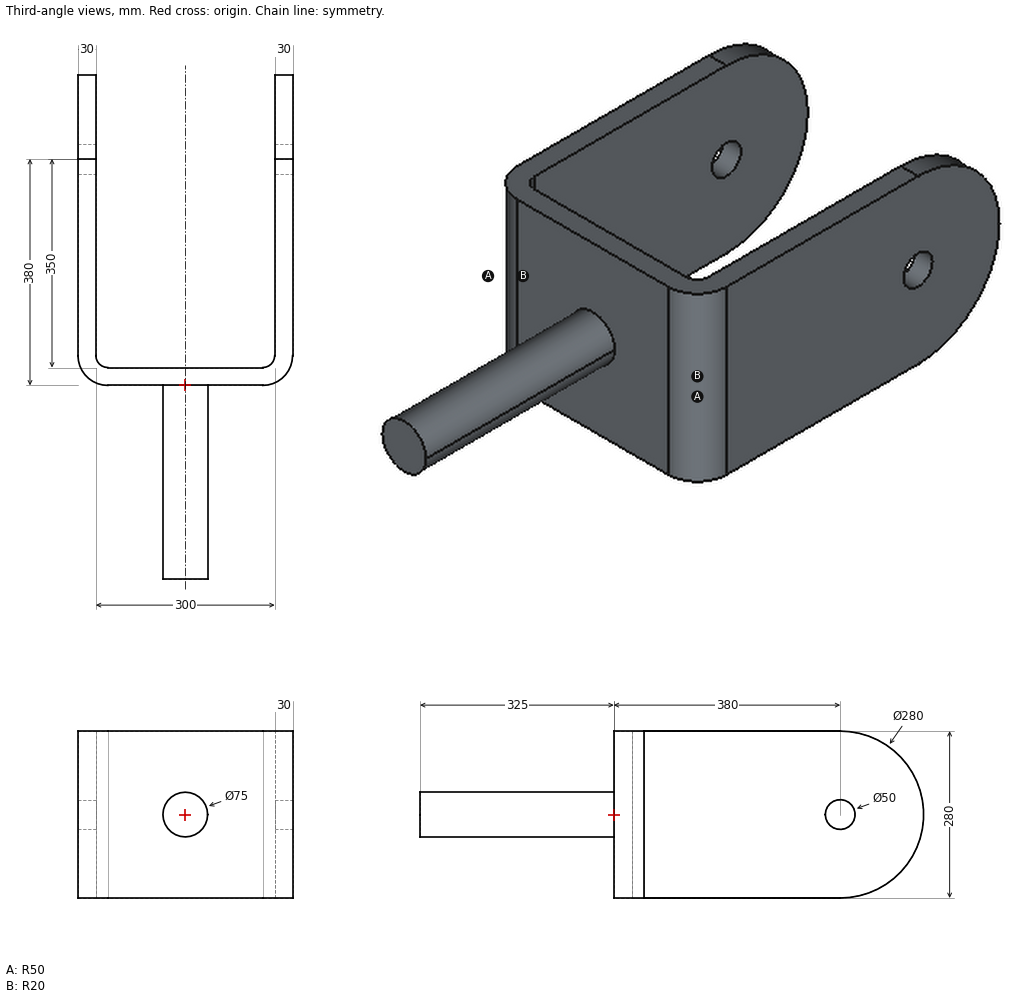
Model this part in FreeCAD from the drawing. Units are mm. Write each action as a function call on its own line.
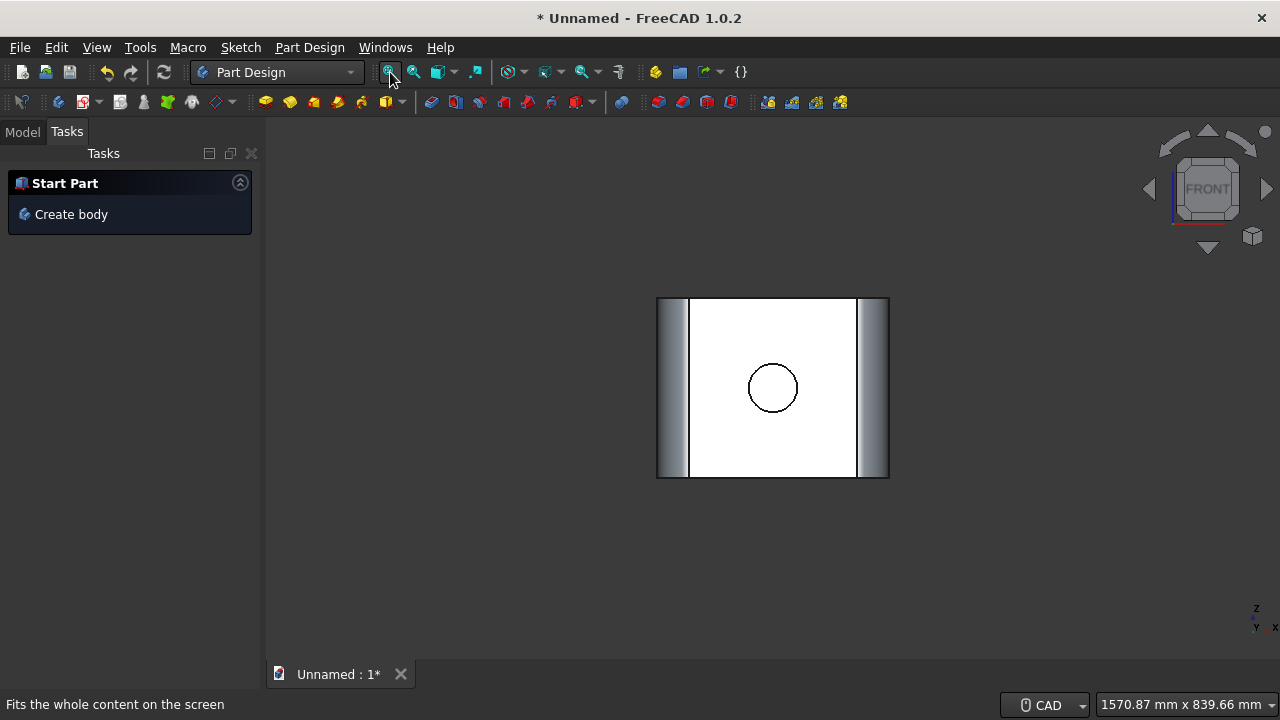
click(390, 72)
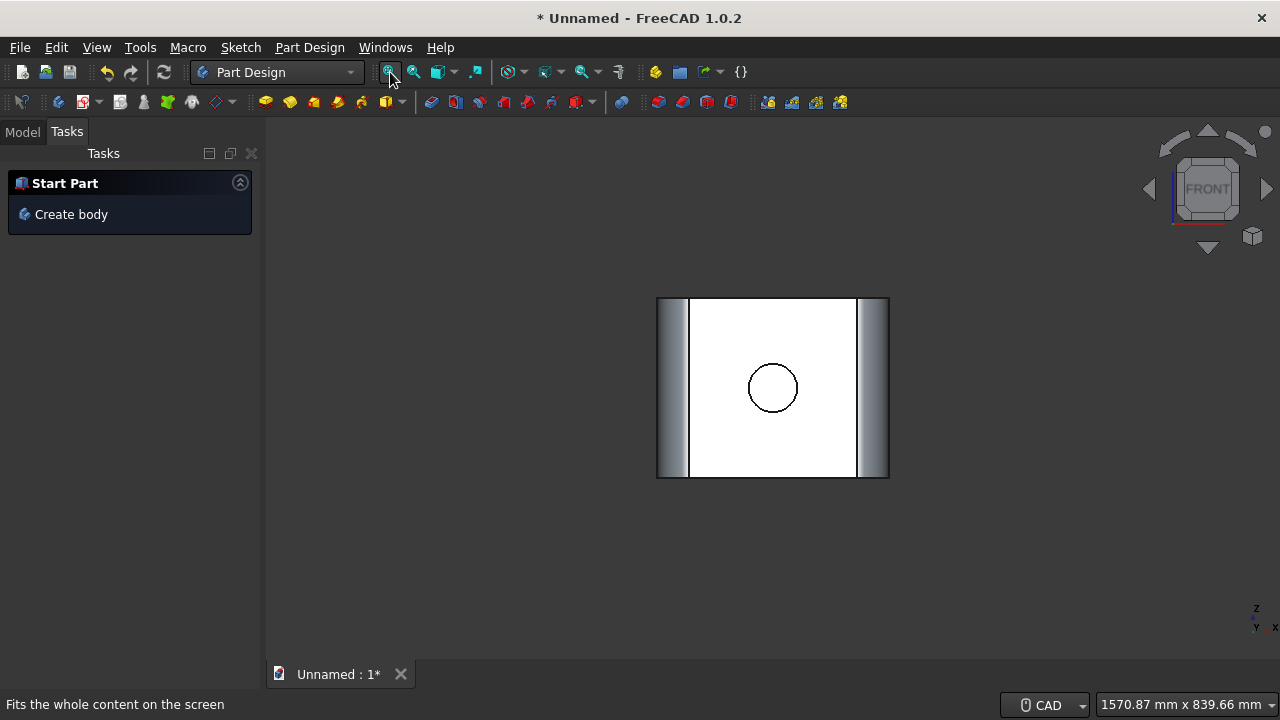
key(3)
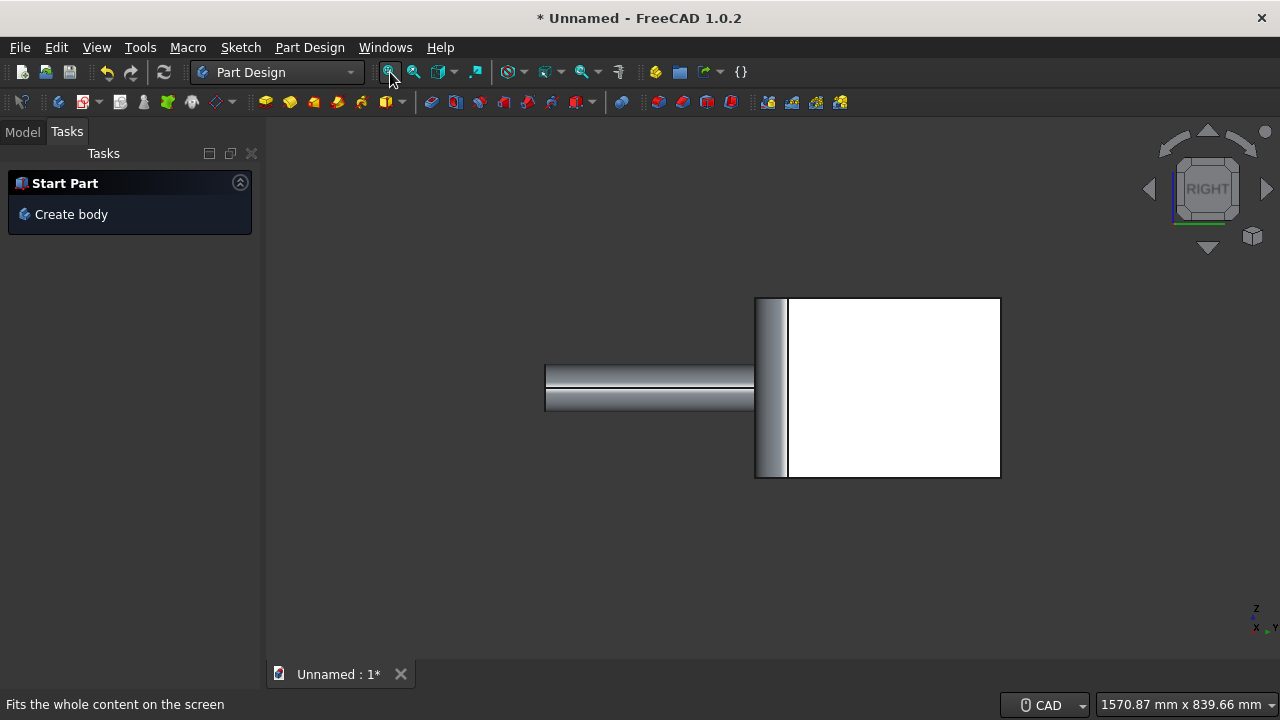
click(390, 72)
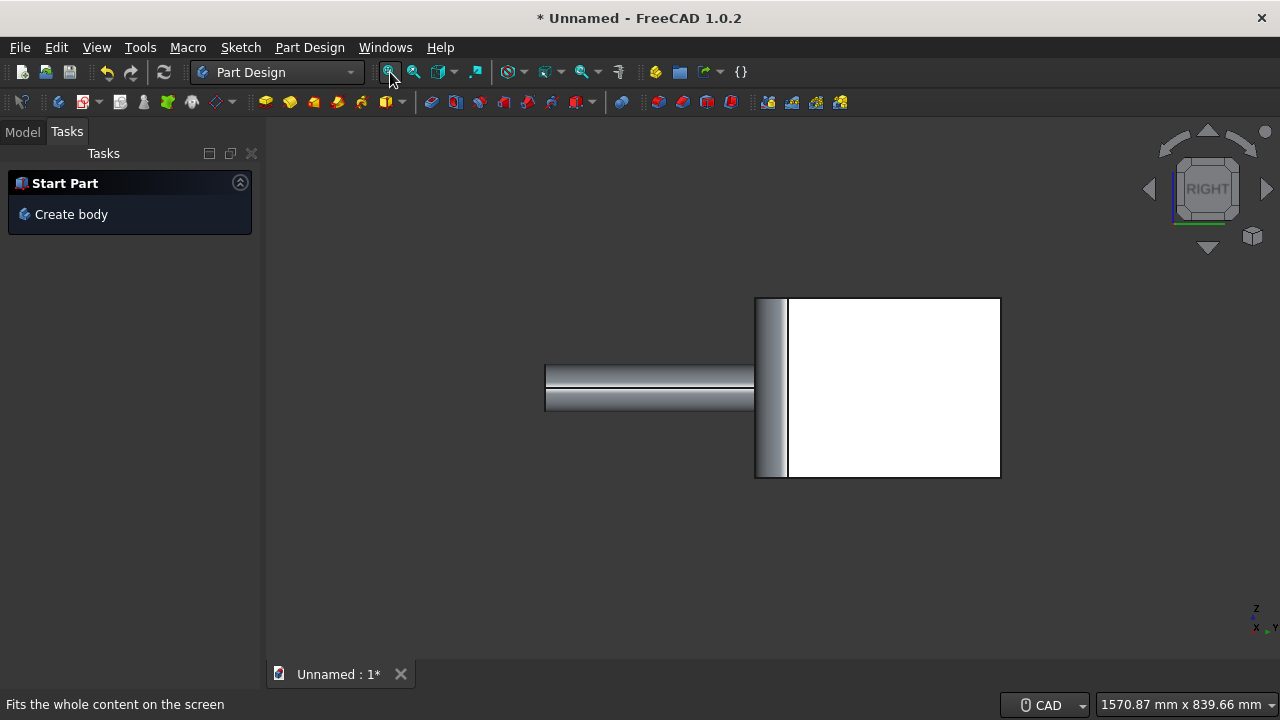
key(5)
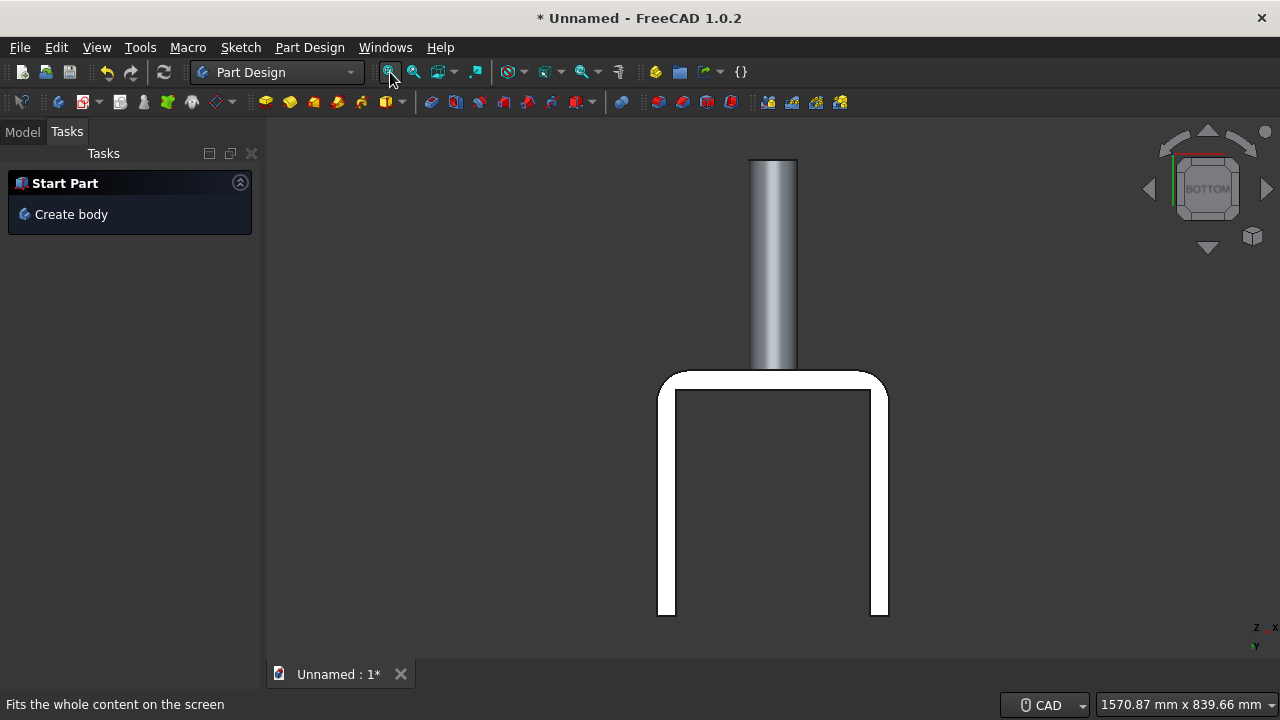
key(4)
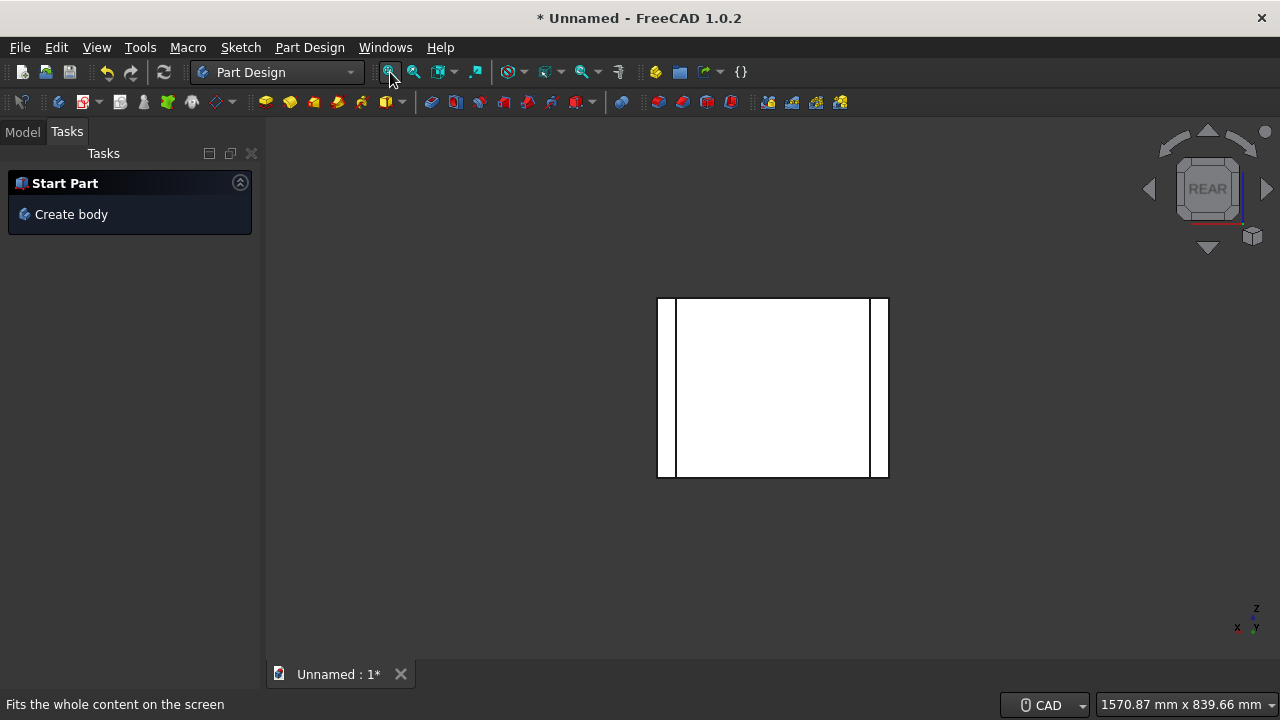
click(390, 72)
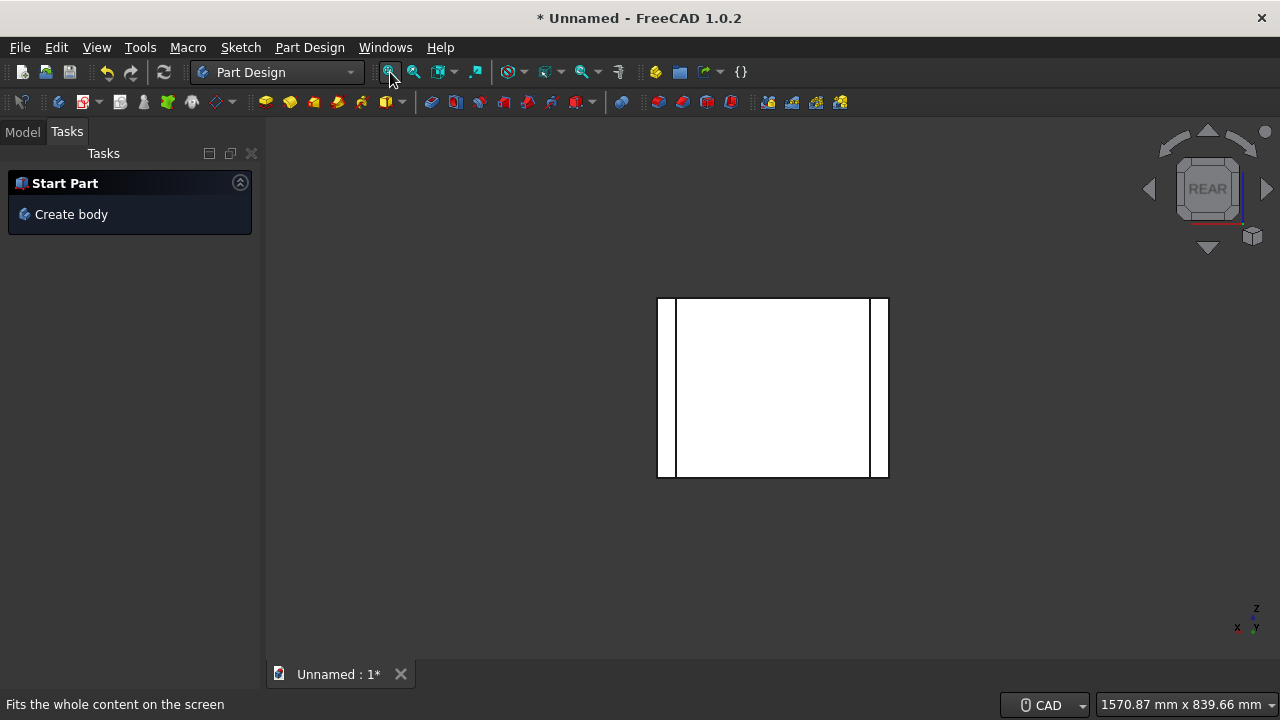
key(6)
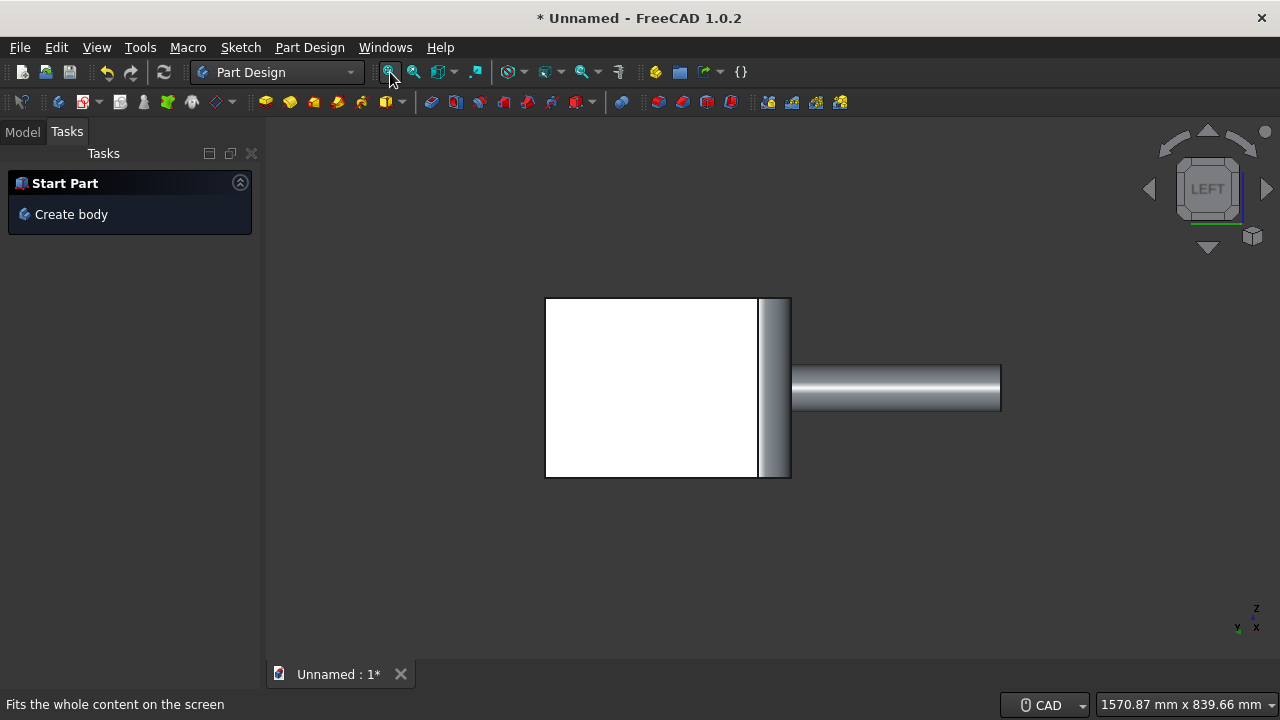
click(390, 72)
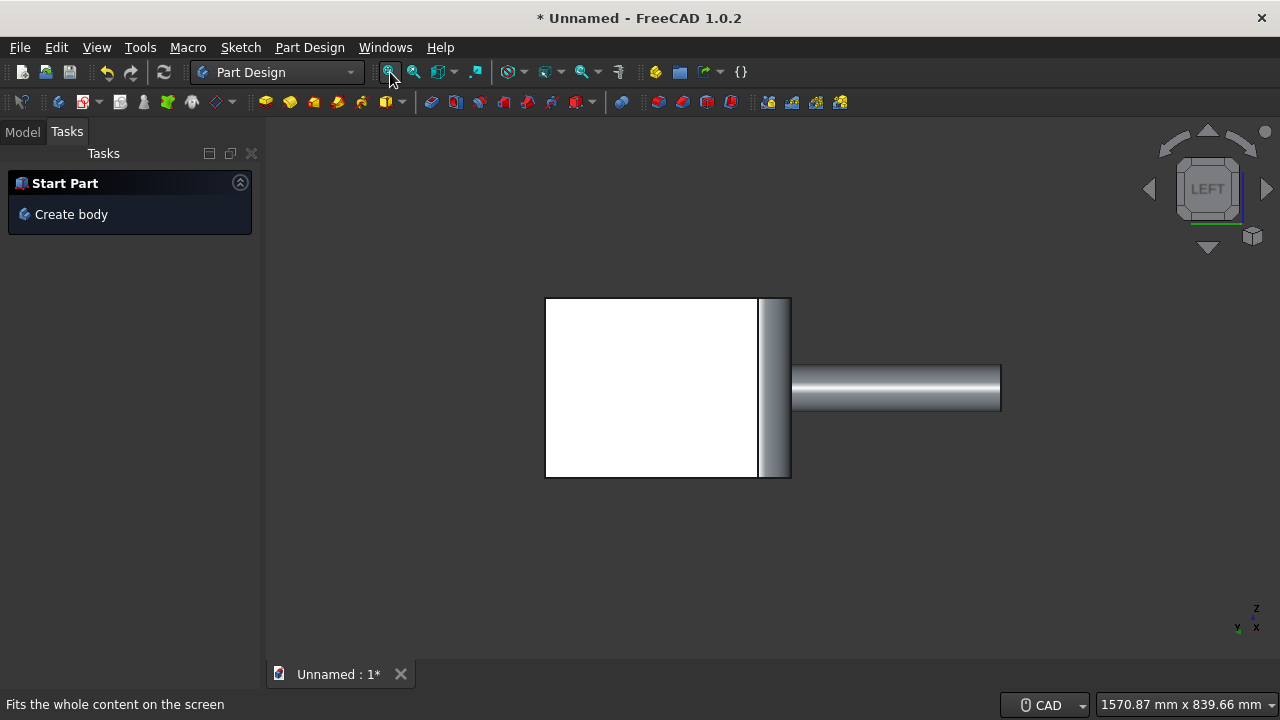
key(v)
key(3)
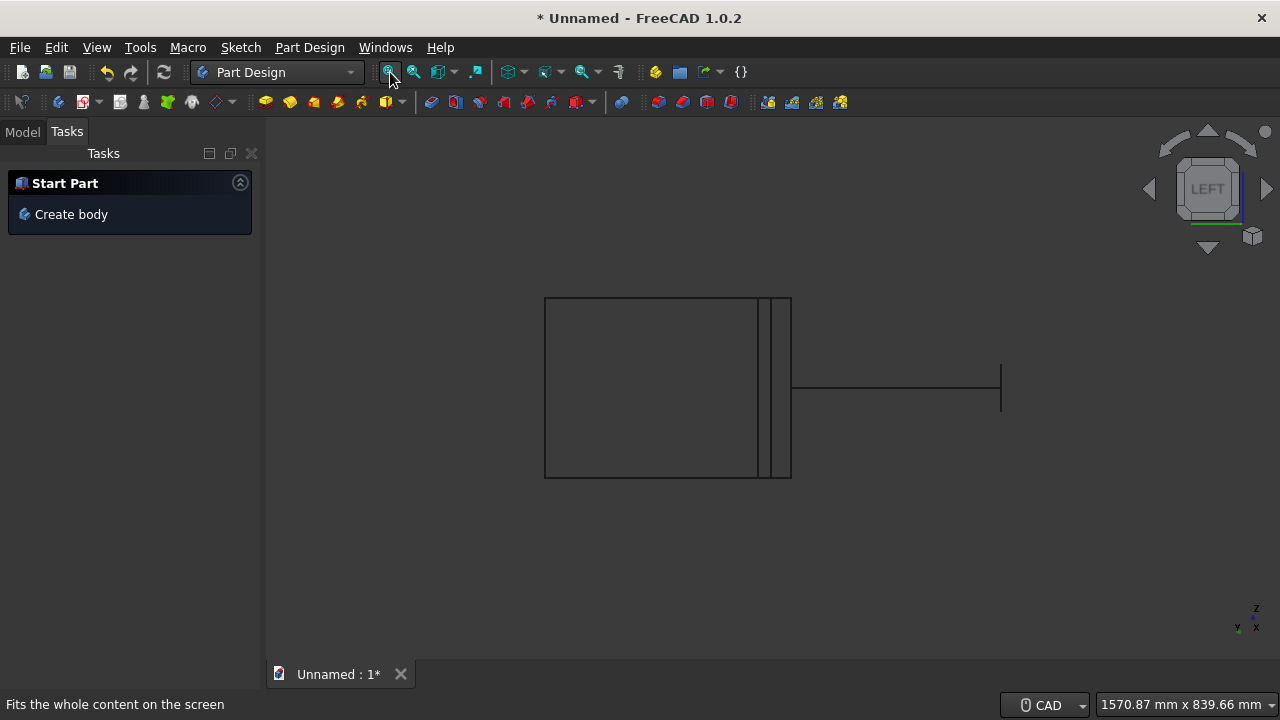
key(0)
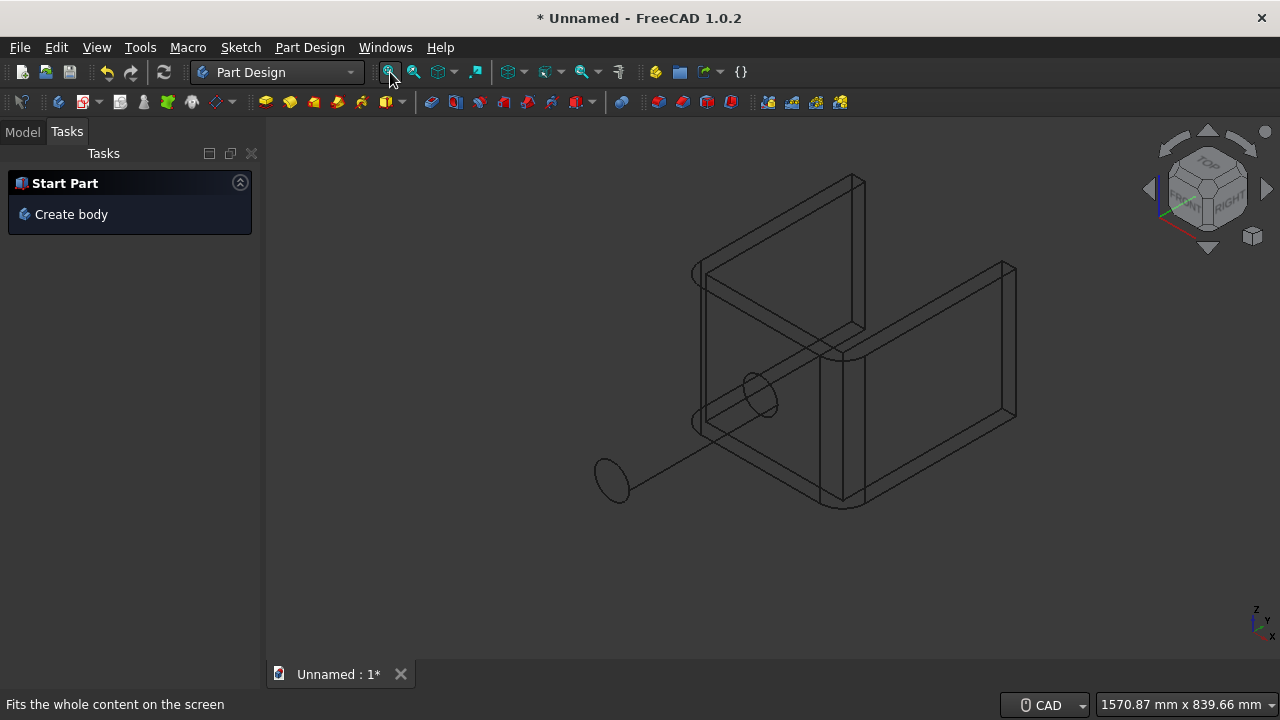
click(843, 426)